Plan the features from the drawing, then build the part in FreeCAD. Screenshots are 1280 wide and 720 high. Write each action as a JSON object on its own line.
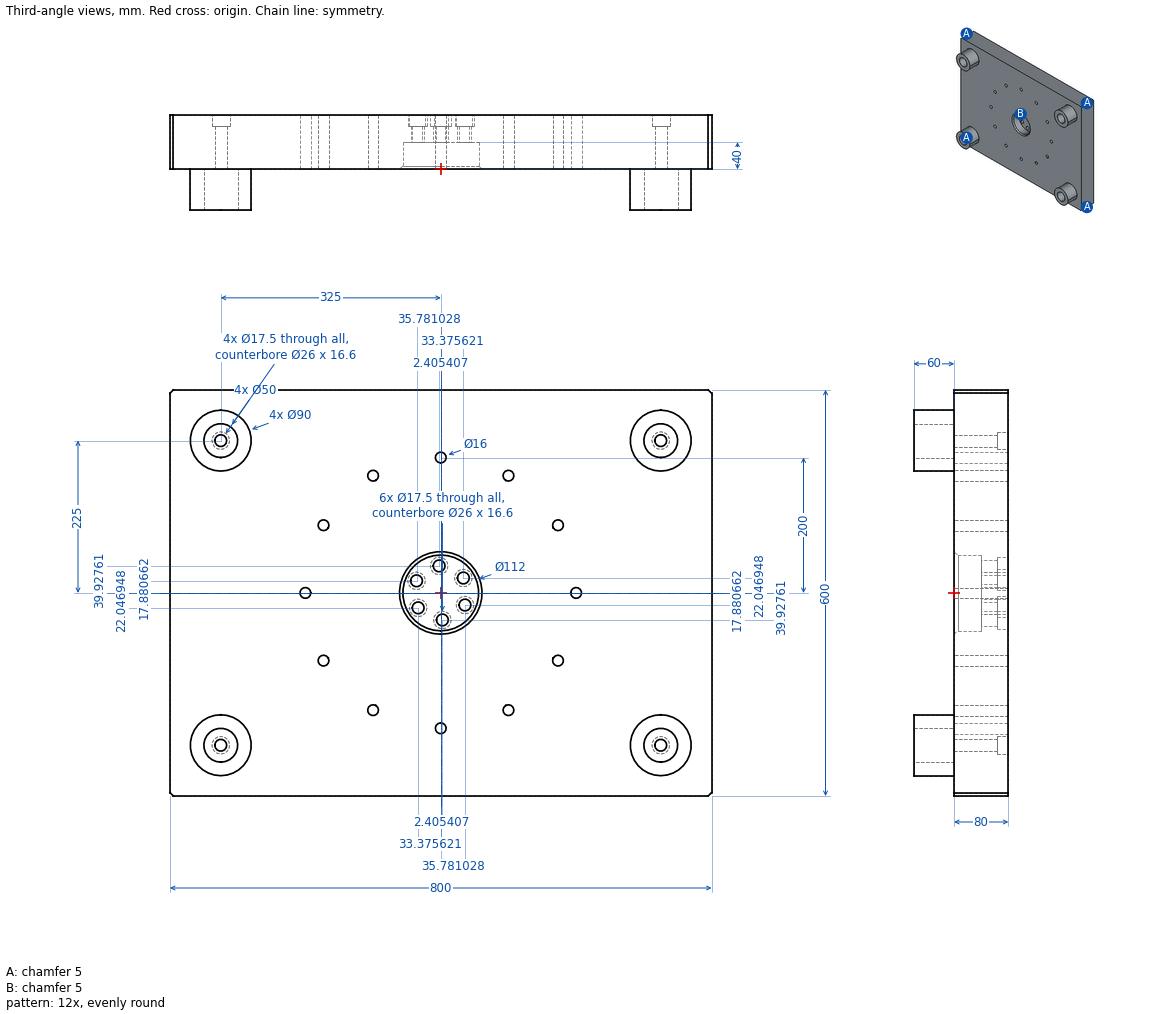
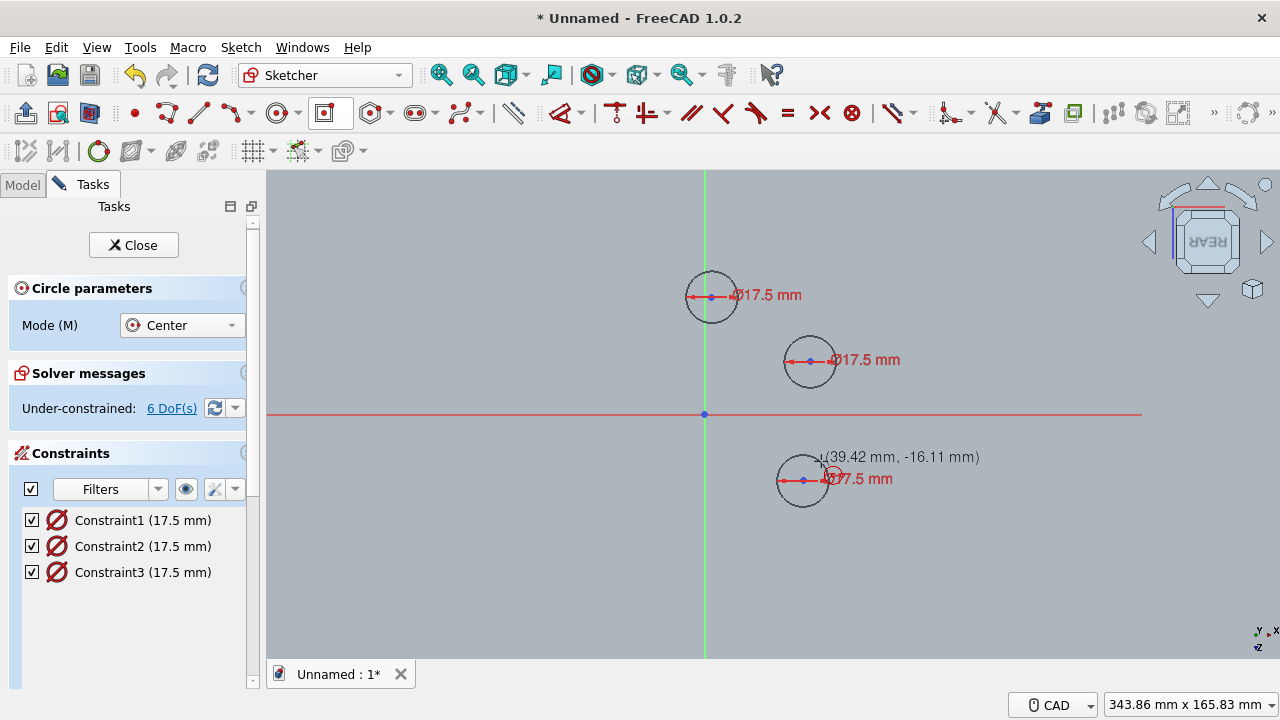
{"action": "scroll", "coordinate": [698, 532], "scroll_direction": "up", "scroll_amount": 5}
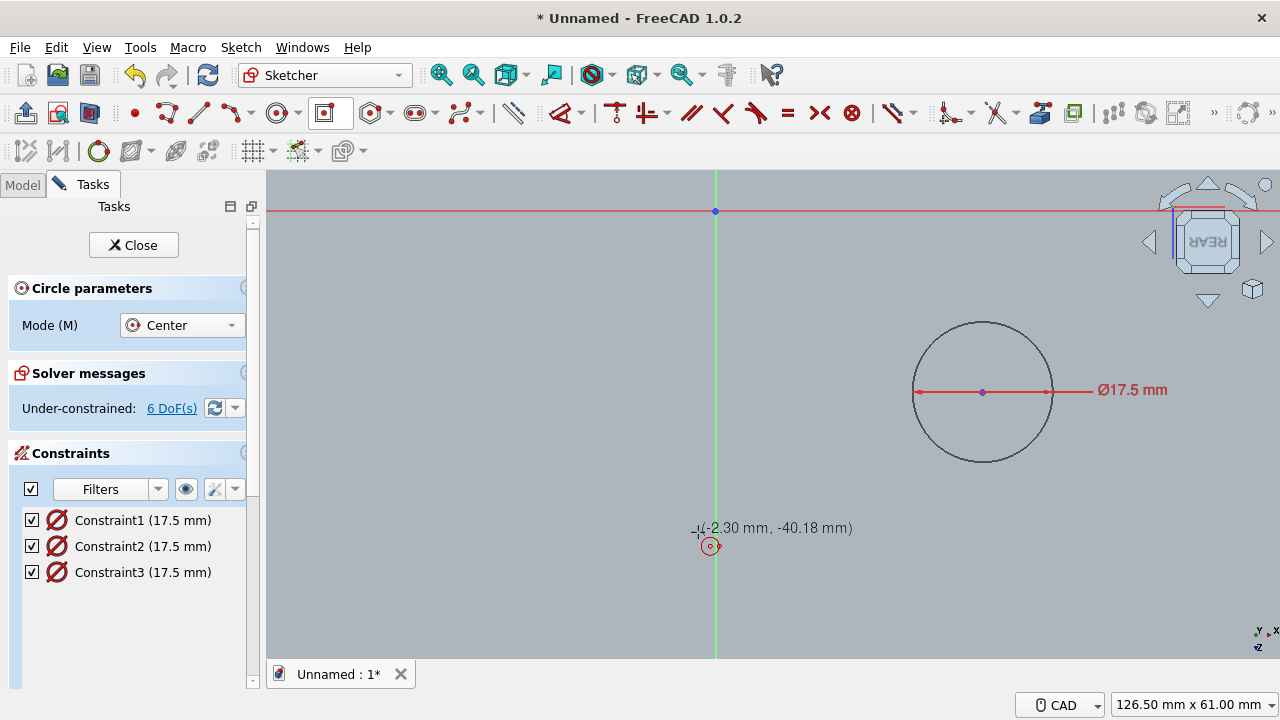
{"action": "left_click", "coordinate": [696, 531]}
{"action": "mouse_move", "coordinate": [746, 482]}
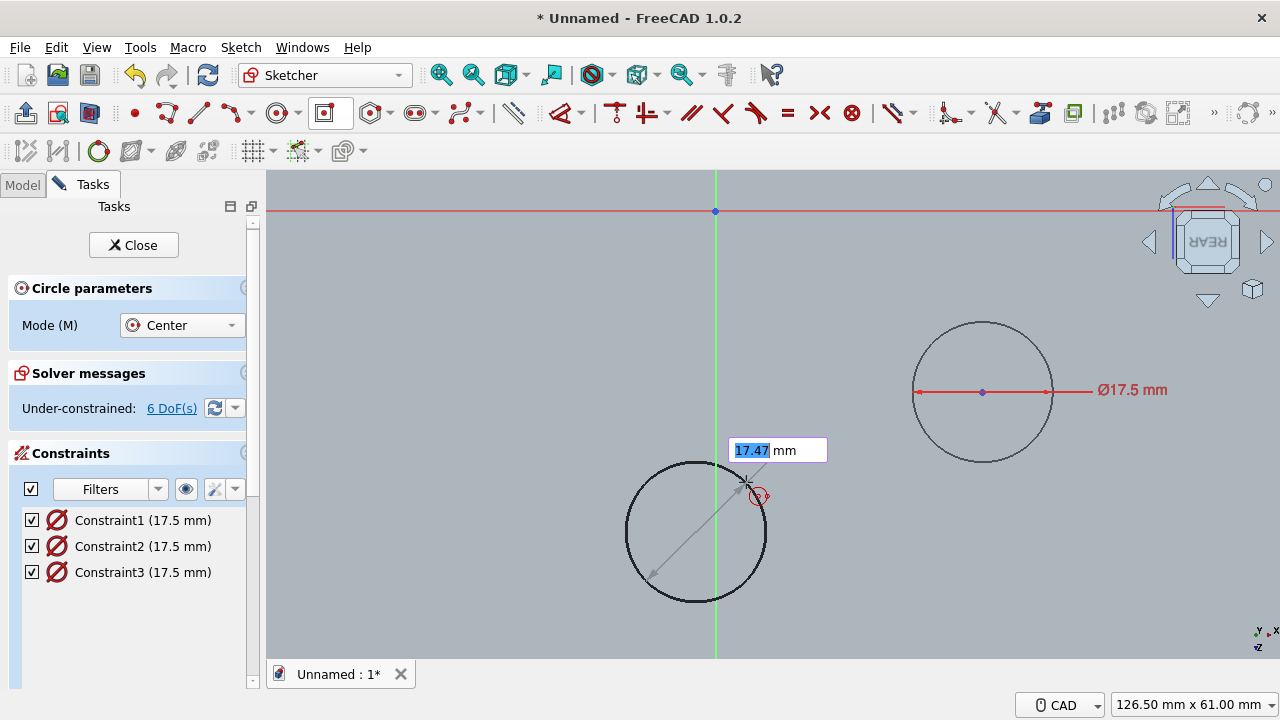
{"action": "type", "text": "17.5"}
{"action": "key", "text": "Return"}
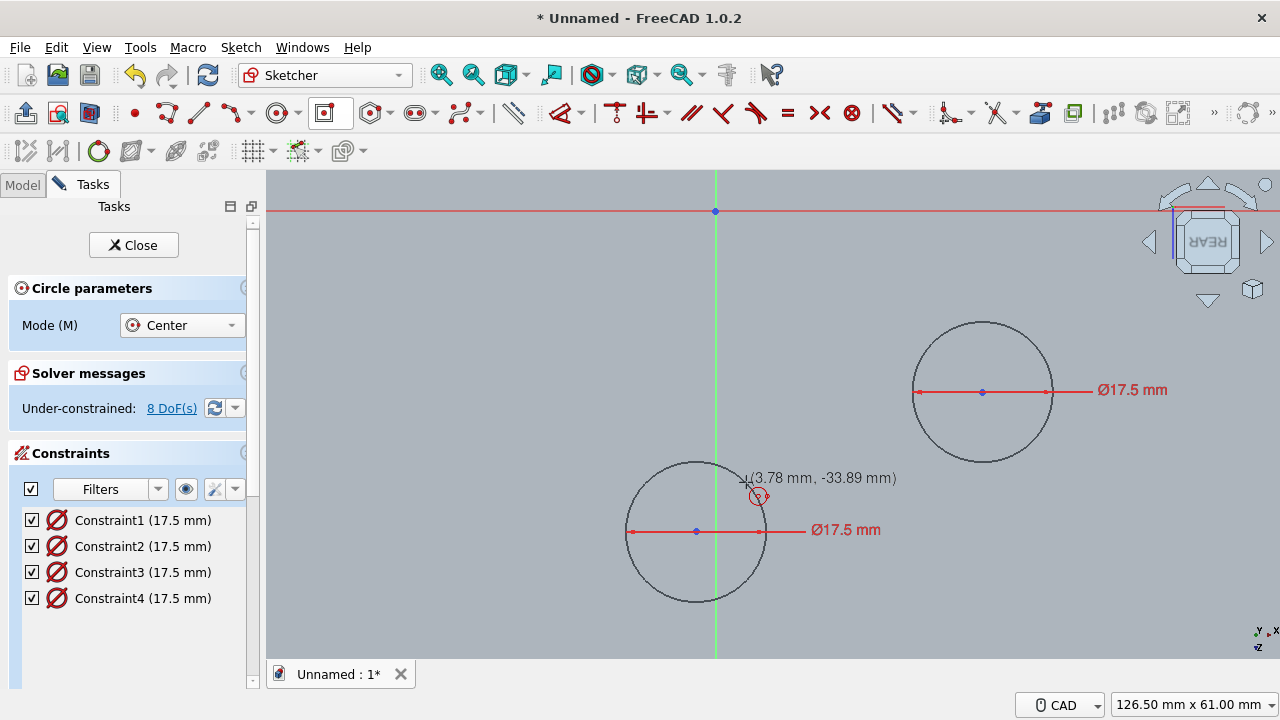
{"action": "left_click", "coordinate": [429, 355]}
{"action": "mouse_move", "coordinate": [478, 305]}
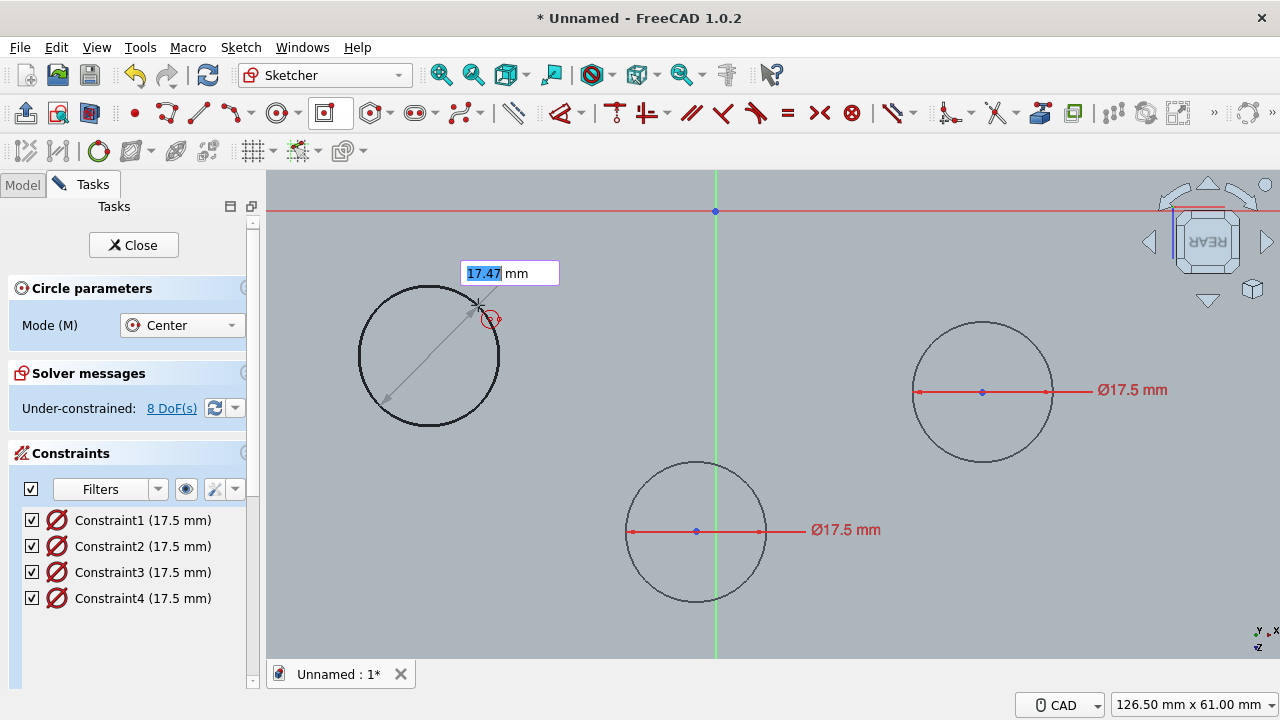
{"action": "type", "text": "17.5"}
{"action": "key", "text": "Return"}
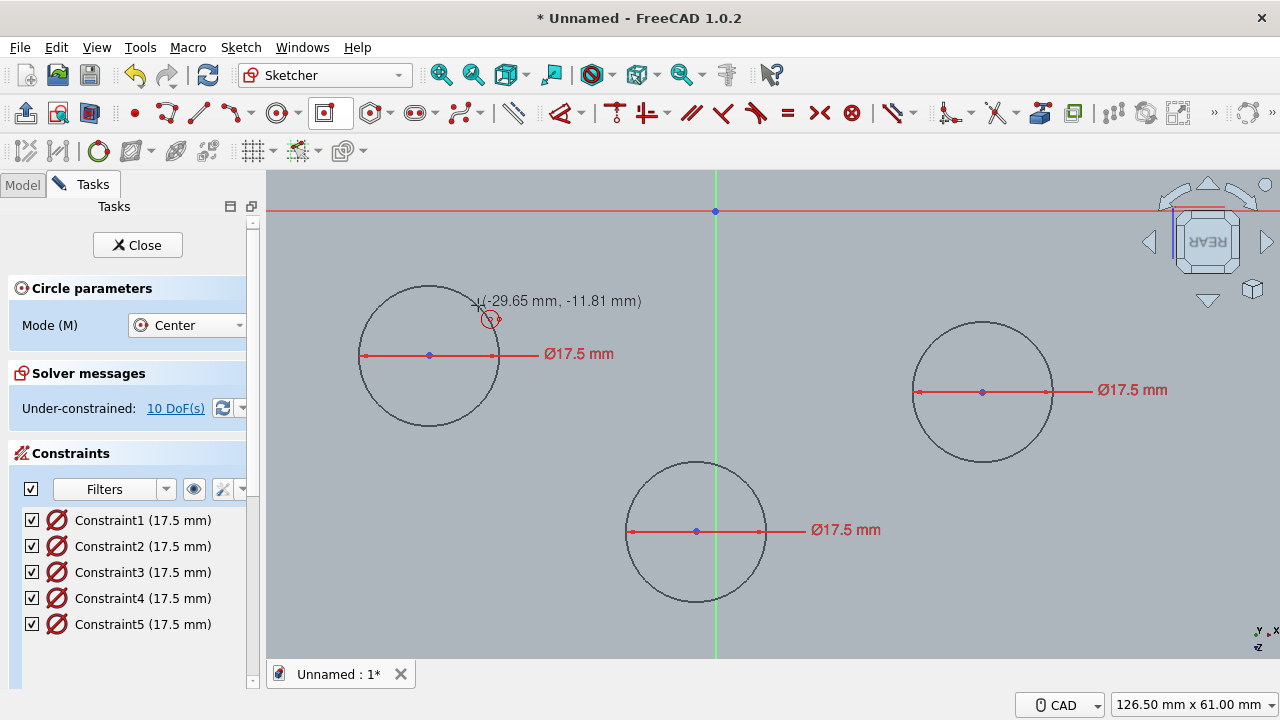
{"action": "scroll", "coordinate": [698, 533], "scroll_direction": "down", "scroll_amount": 5}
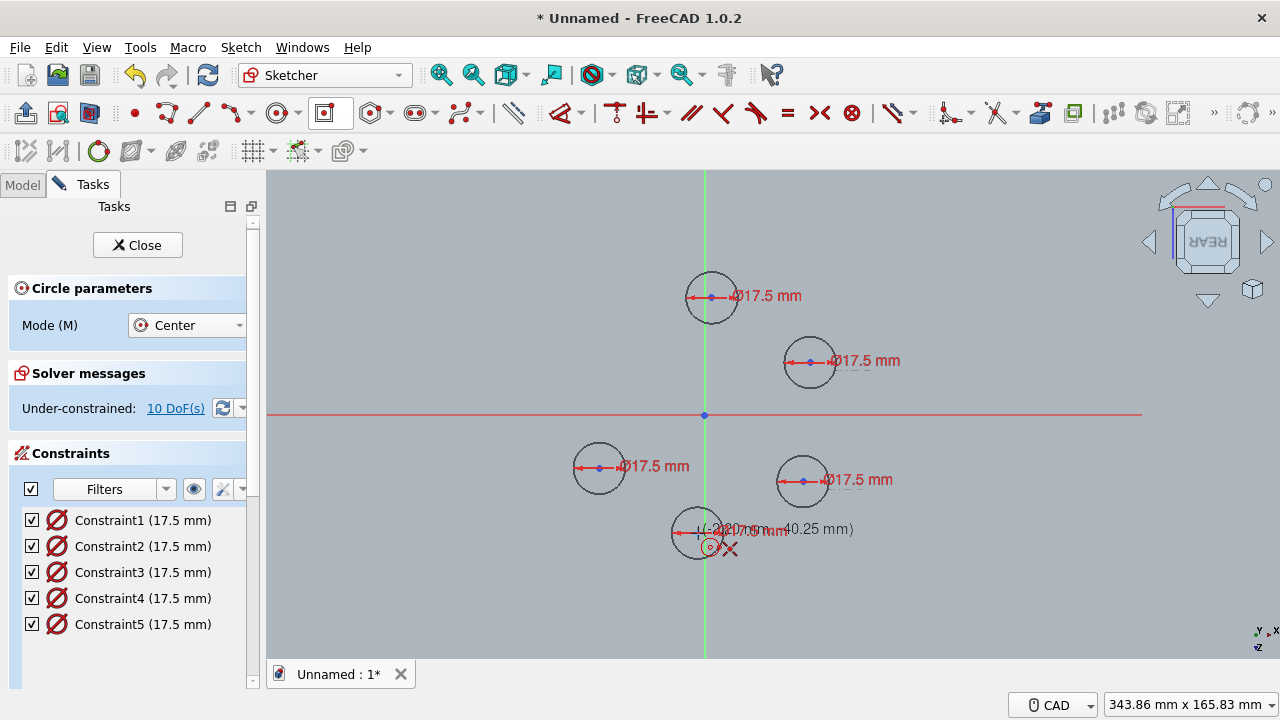
{"action": "left_click", "coordinate": [606, 350]}
{"action": "mouse_move", "coordinate": [625, 332]}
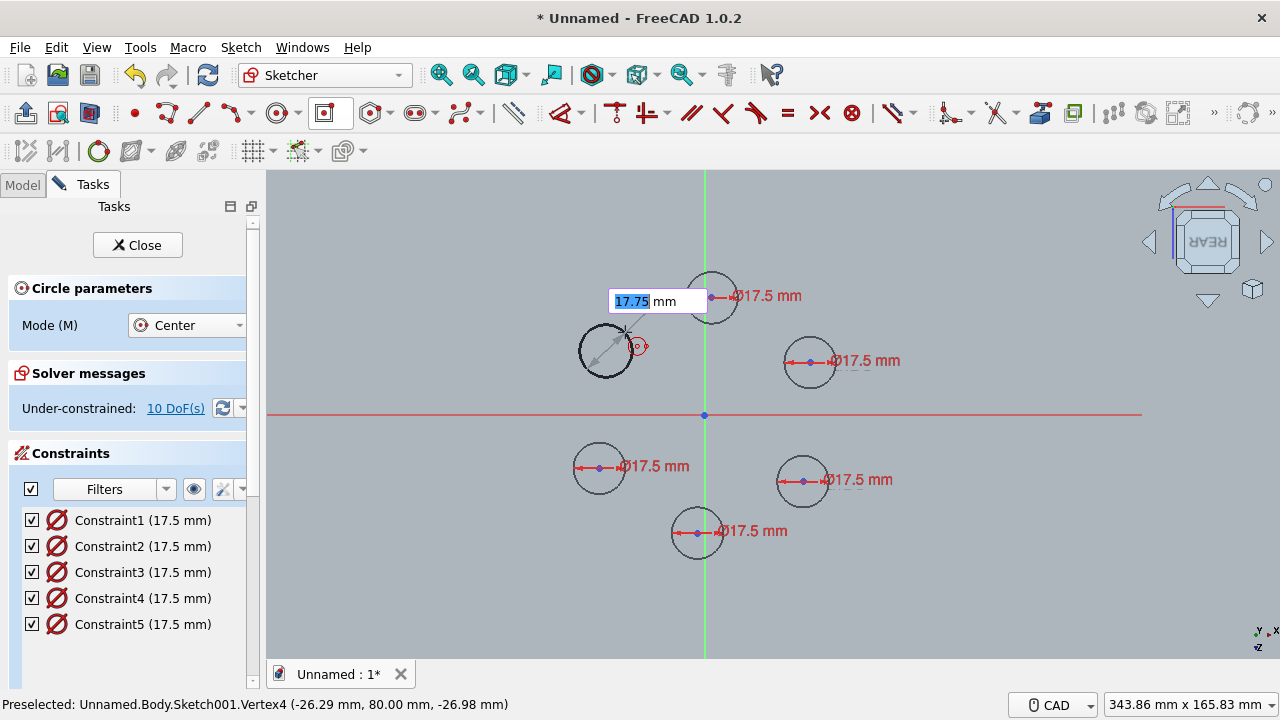
{"action": "type", "text": "17.5"}
{"action": "key", "text": "Return"}
{"action": "key", "text": "Escape"}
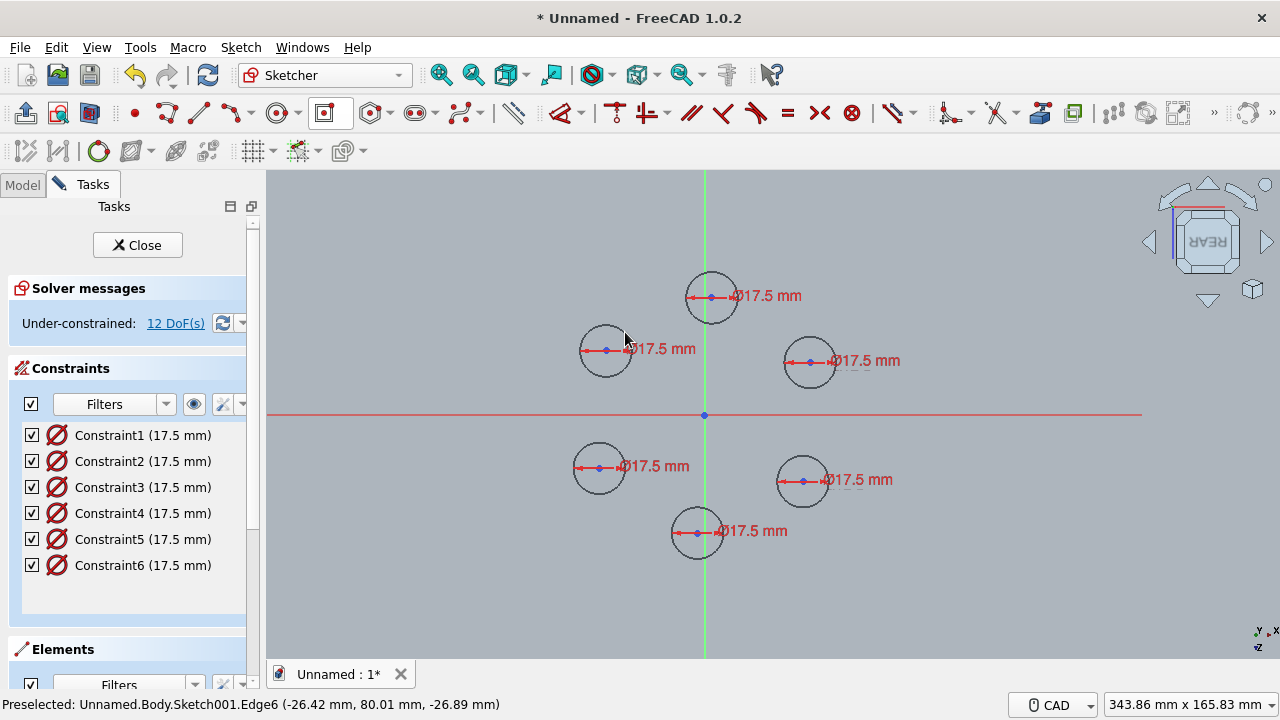
{"action": "scroll", "coordinate": [712, 298], "scroll_direction": "up", "scroll_amount": 9}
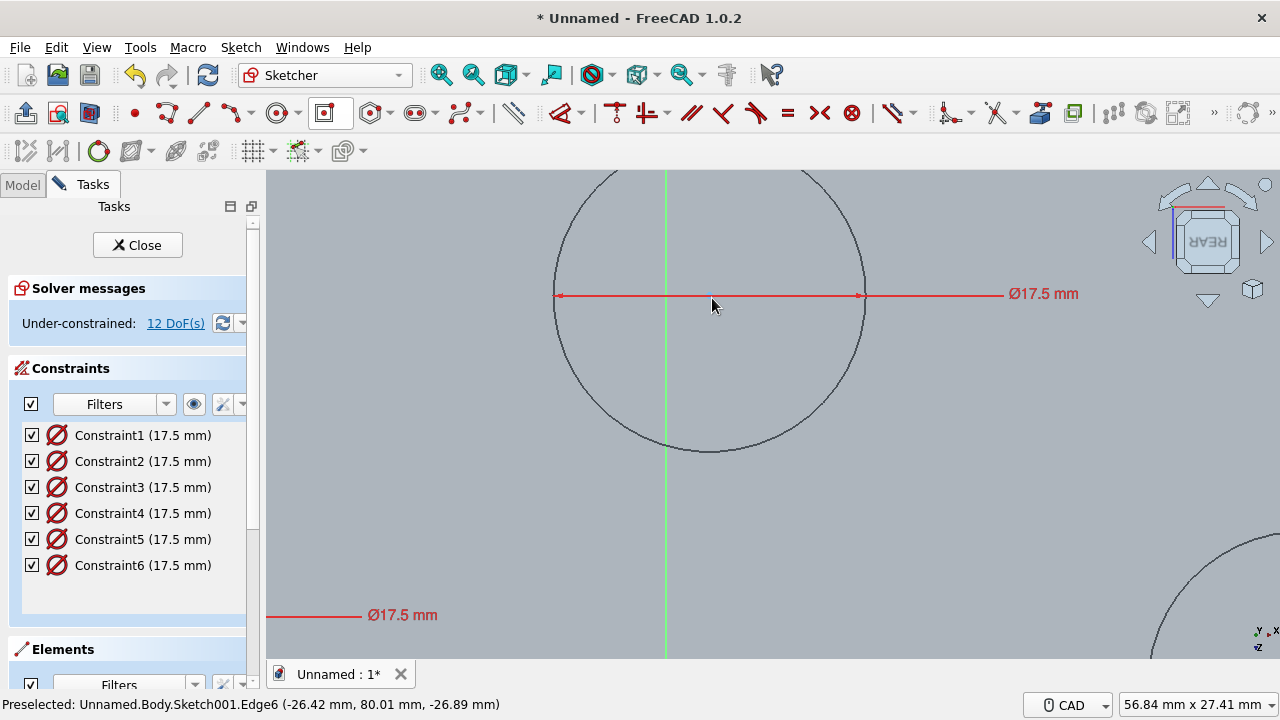
{"action": "left_click", "coordinate": [710, 296]}